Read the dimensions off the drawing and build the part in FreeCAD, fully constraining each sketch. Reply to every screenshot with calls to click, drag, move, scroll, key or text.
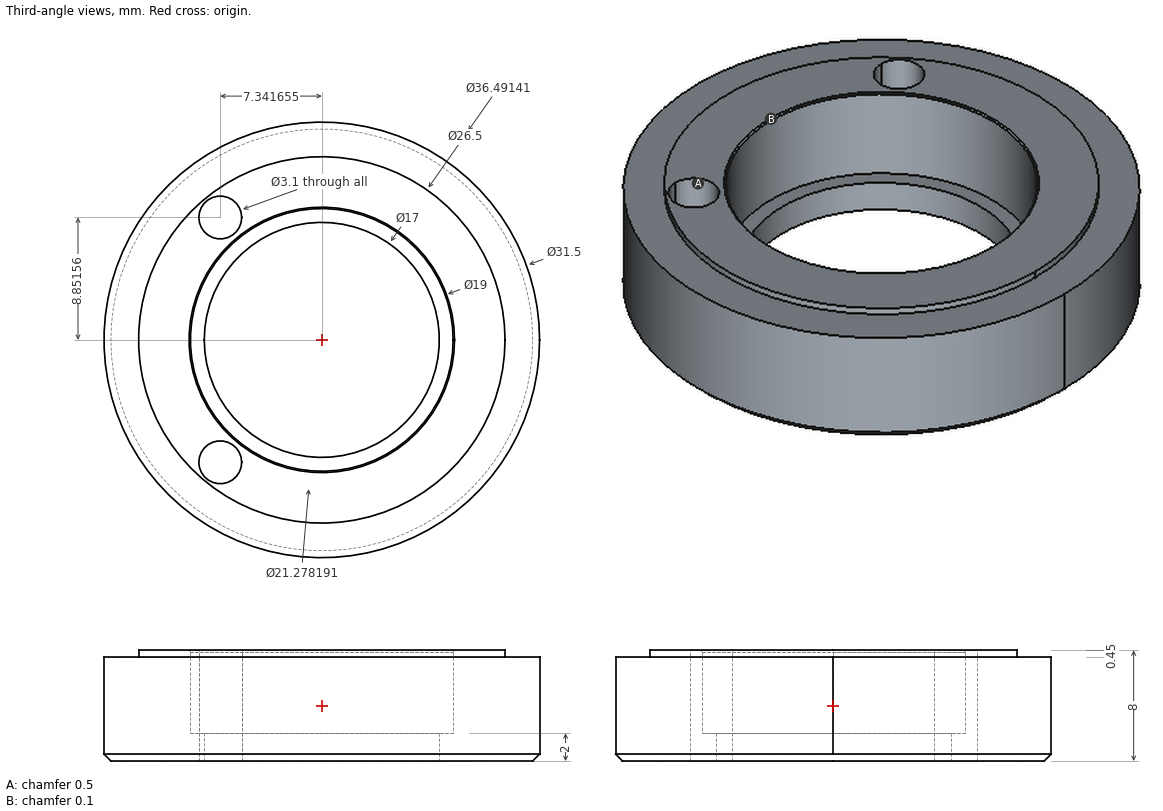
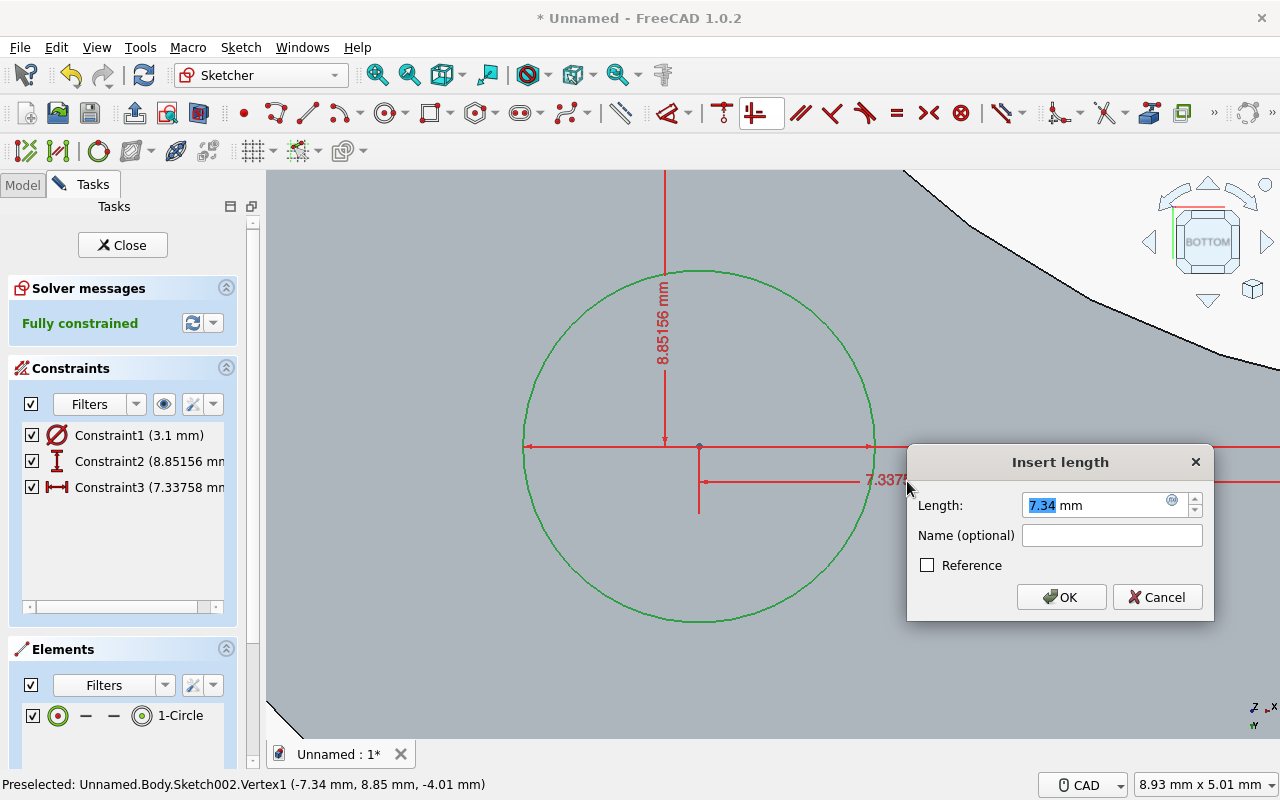
text(7.341655)
key(Return)
key(Escape)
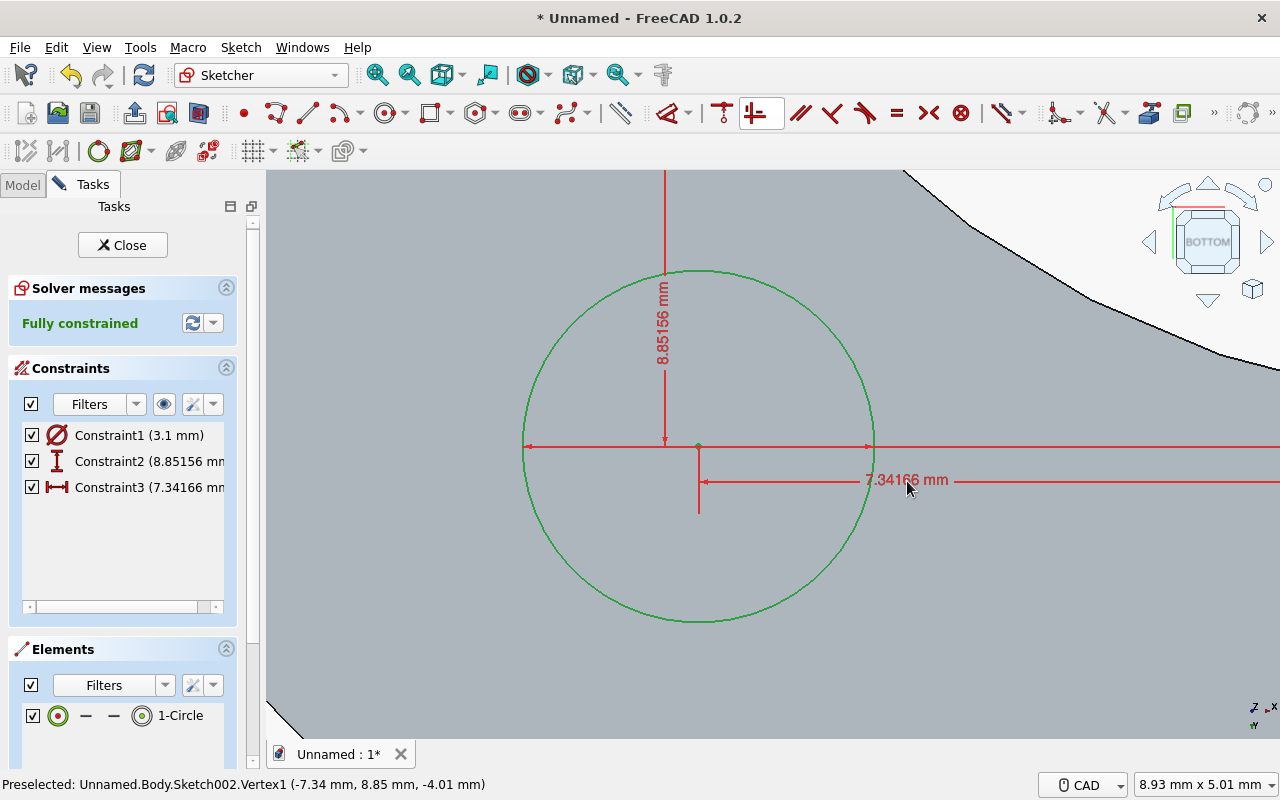
click(123, 245)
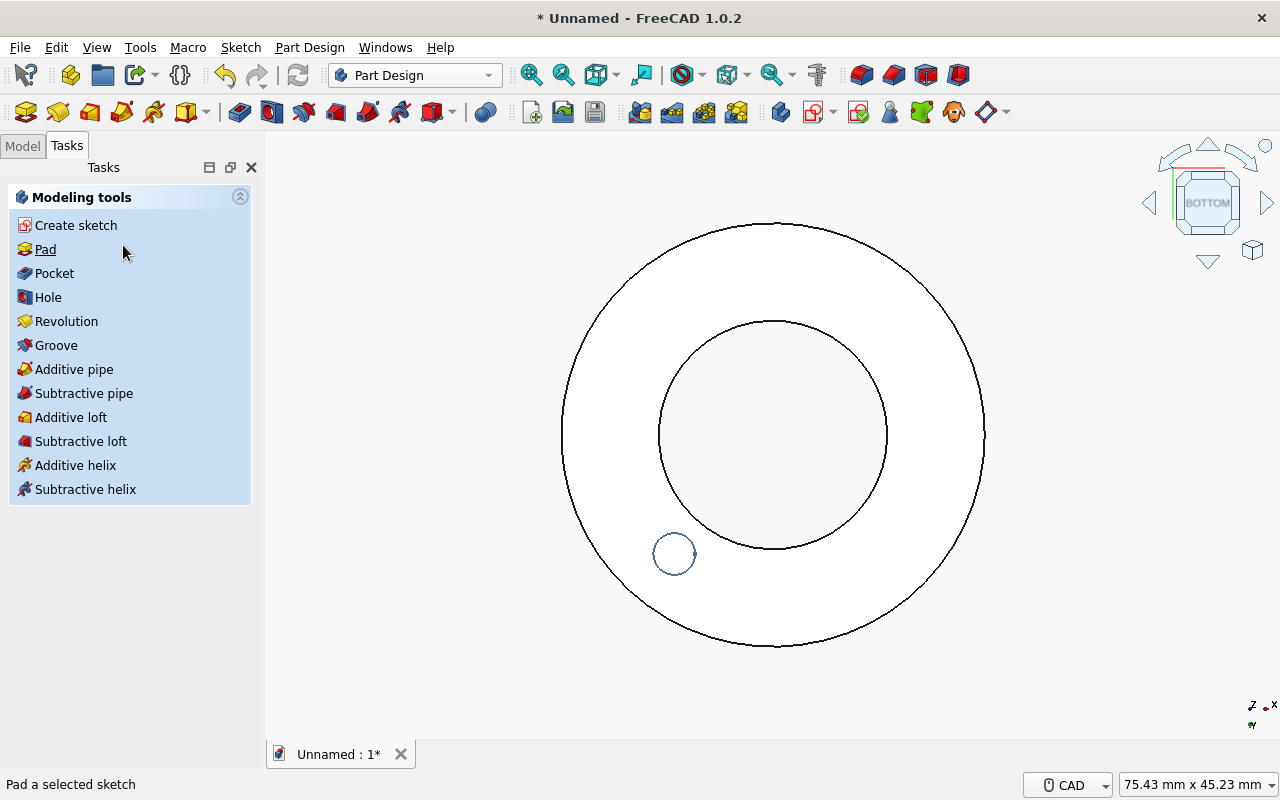
click(272, 112)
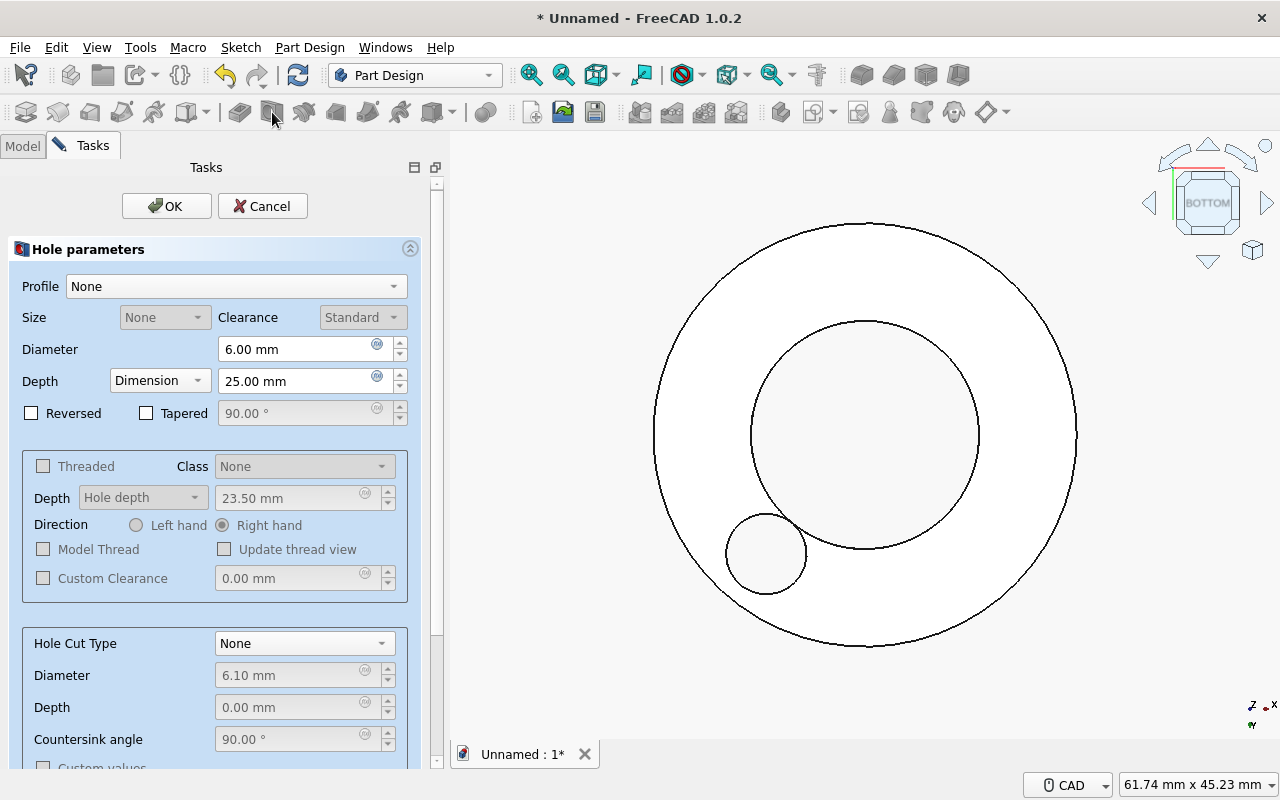
triple_click(305, 349)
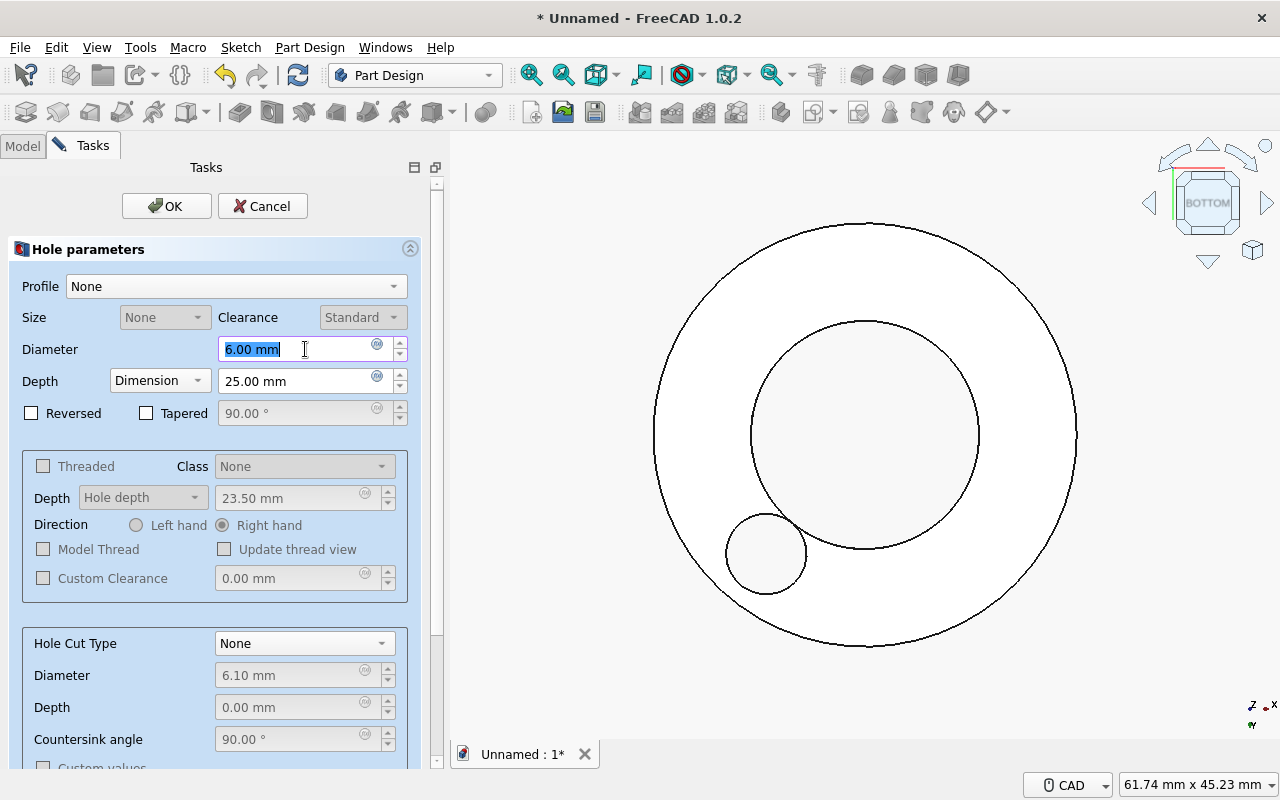
text(3.1)
key(Tab)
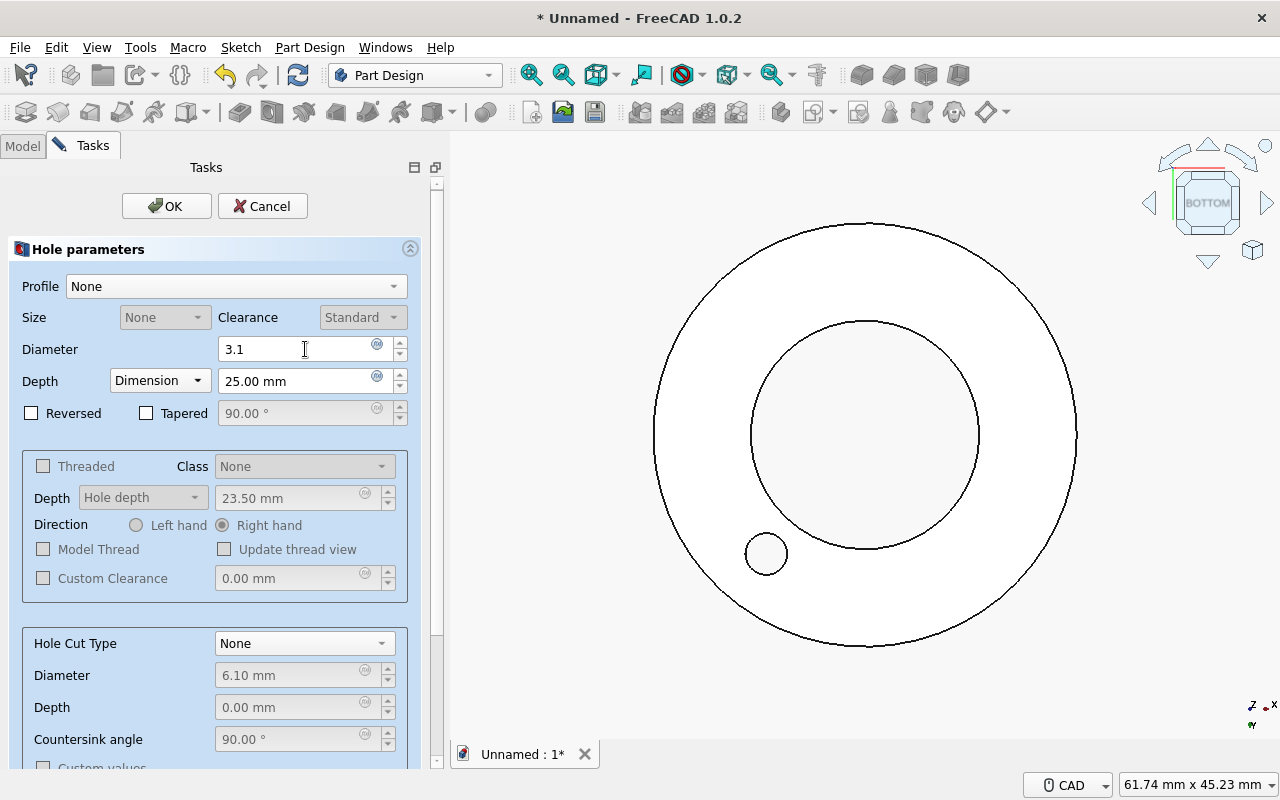
click(161, 380)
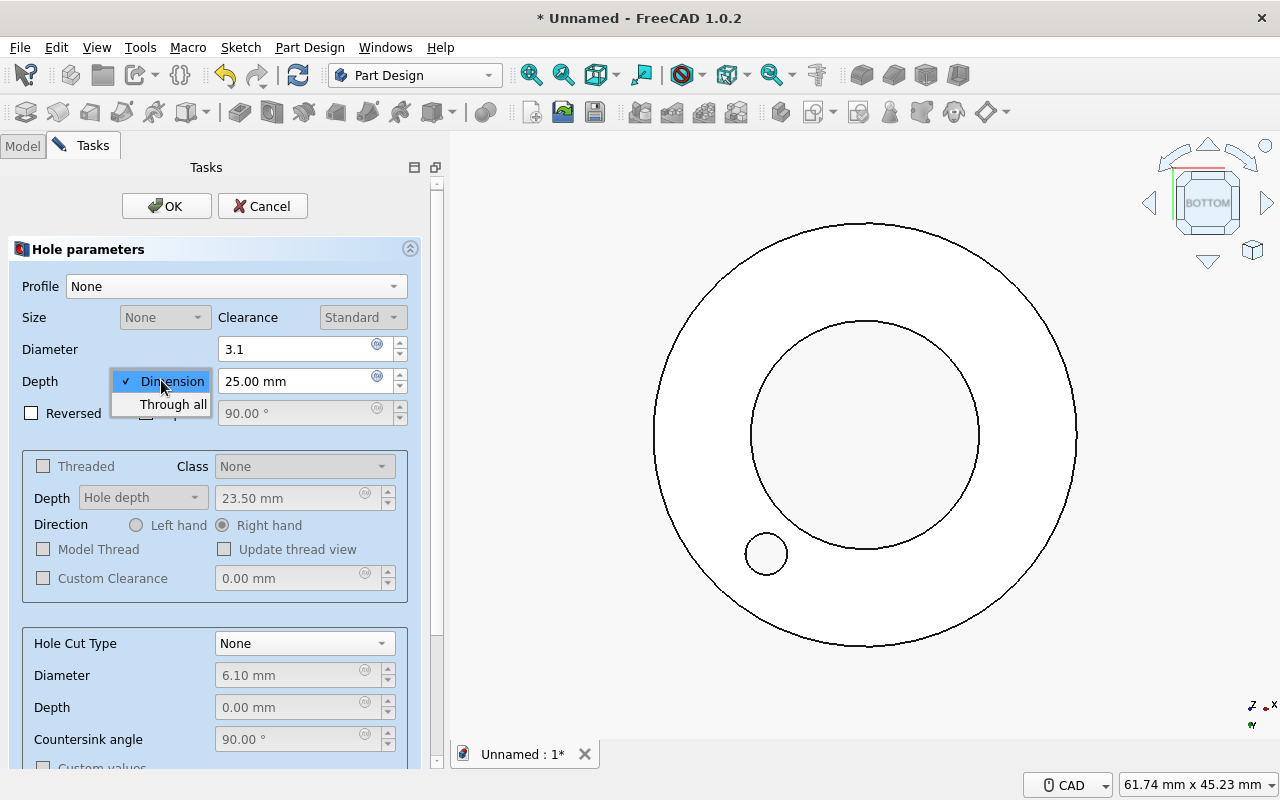
click(160, 404)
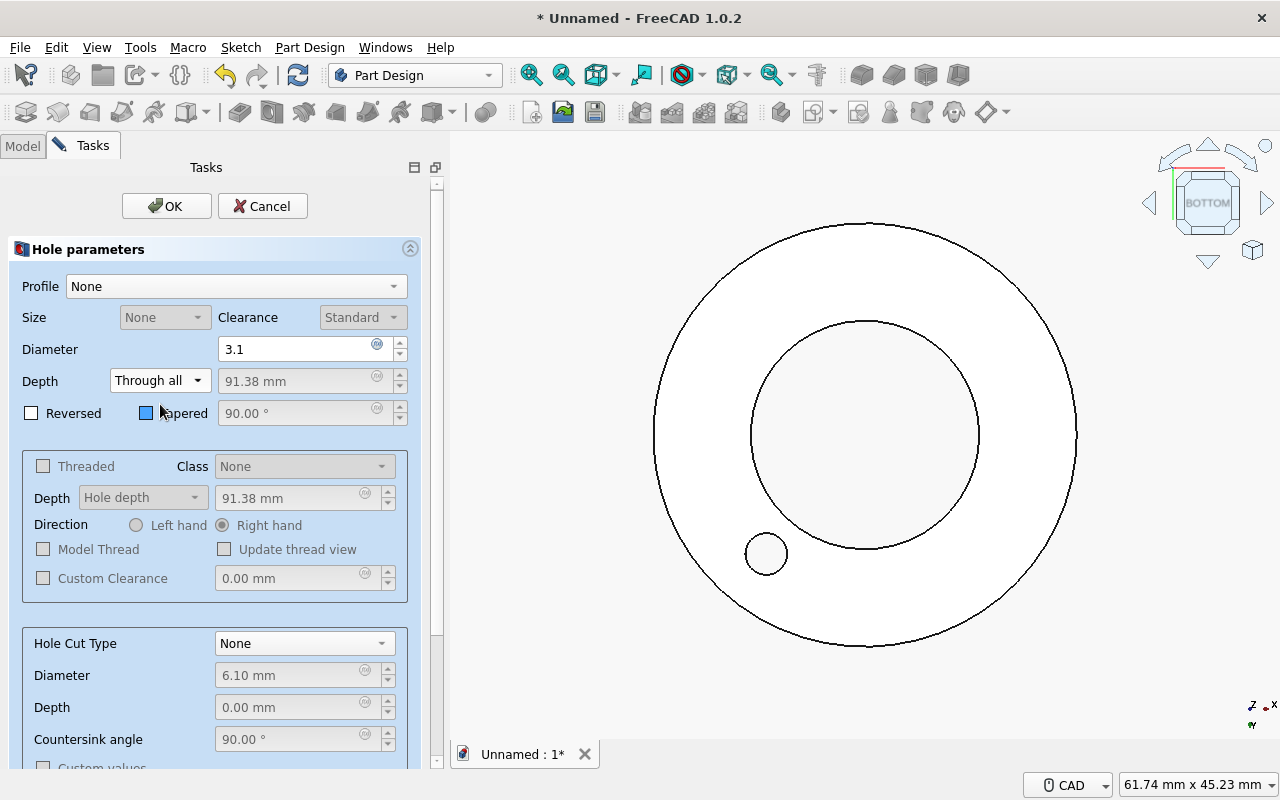
click(167, 206)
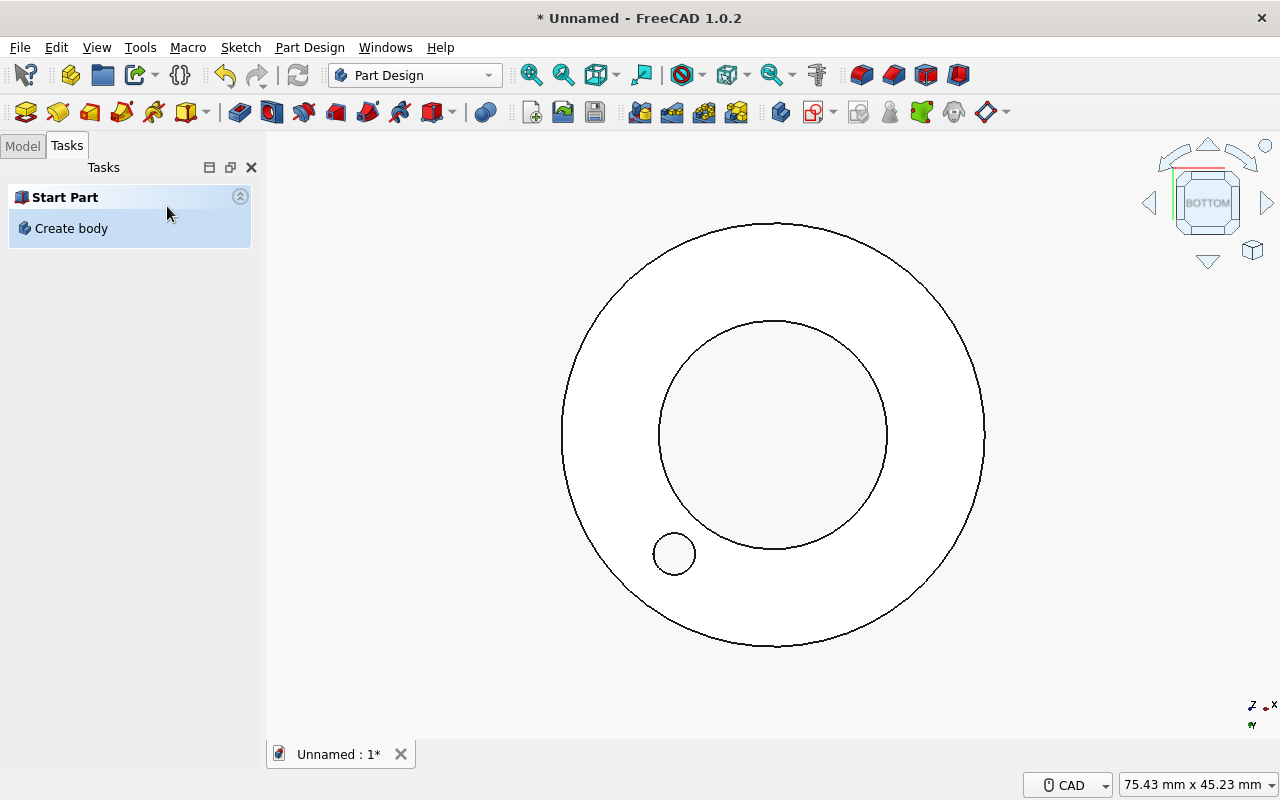
click(23, 145)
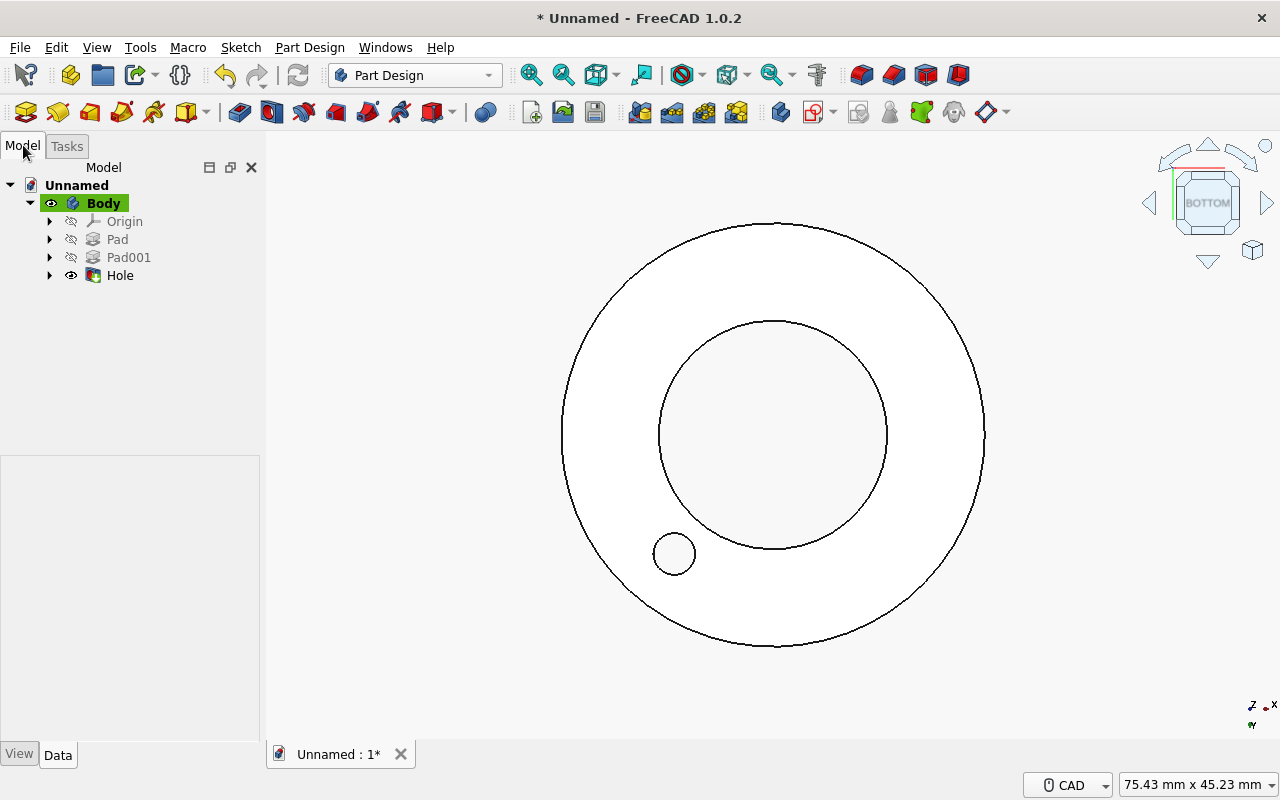
click(116, 275)